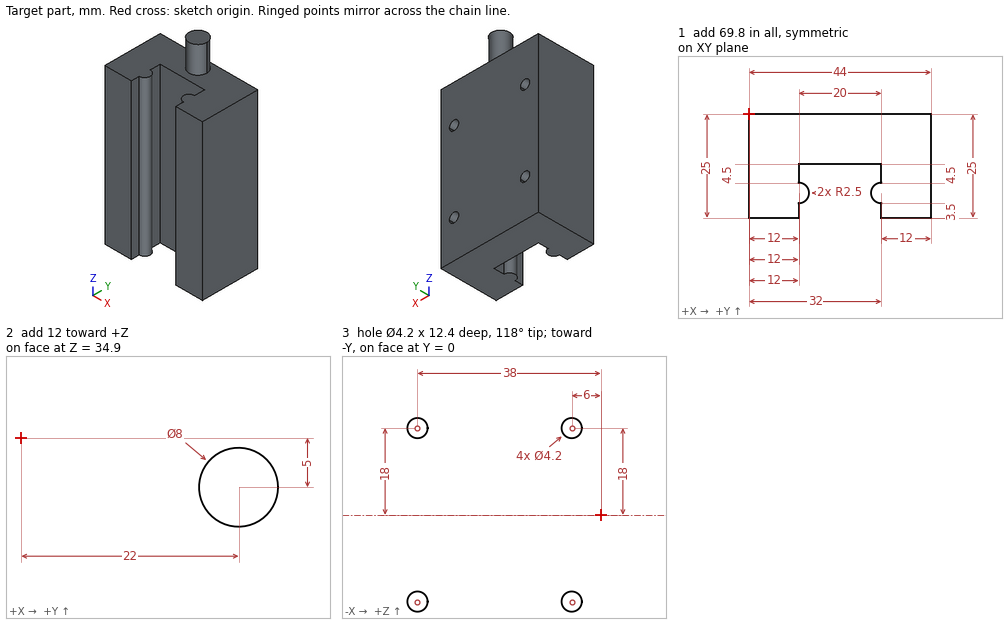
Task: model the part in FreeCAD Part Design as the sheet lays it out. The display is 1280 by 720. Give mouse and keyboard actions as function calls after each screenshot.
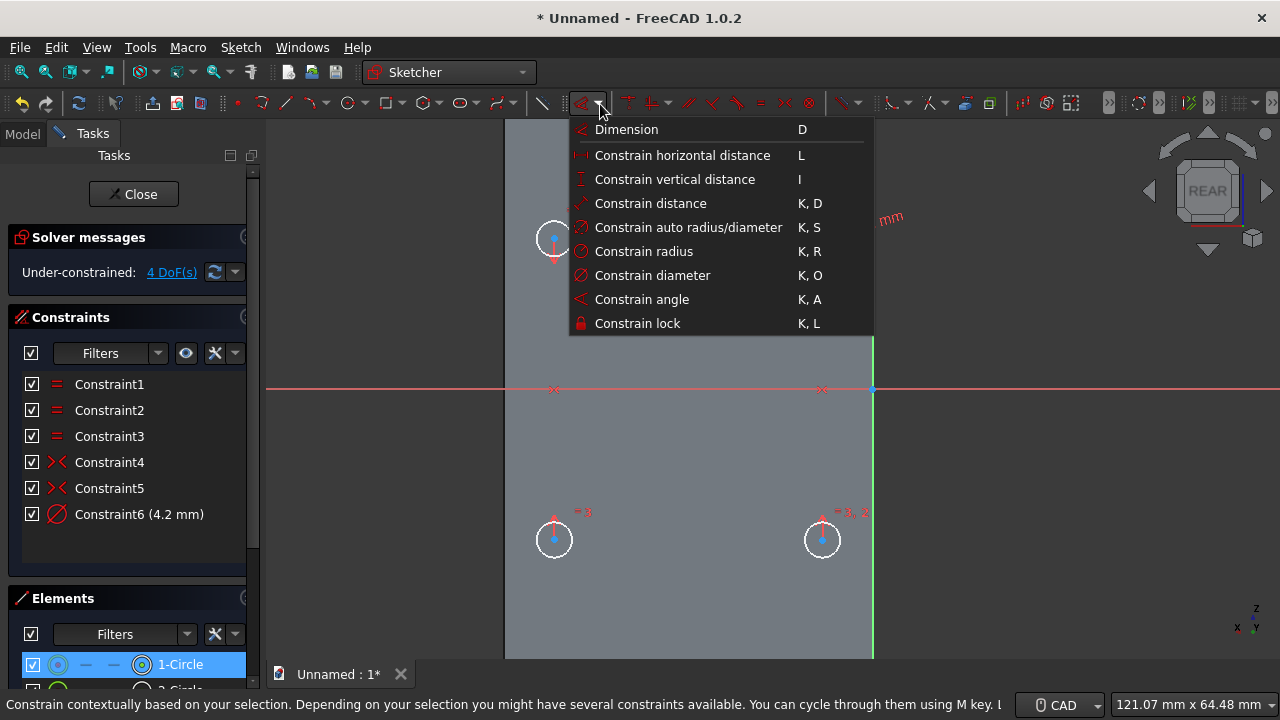
click(722, 155)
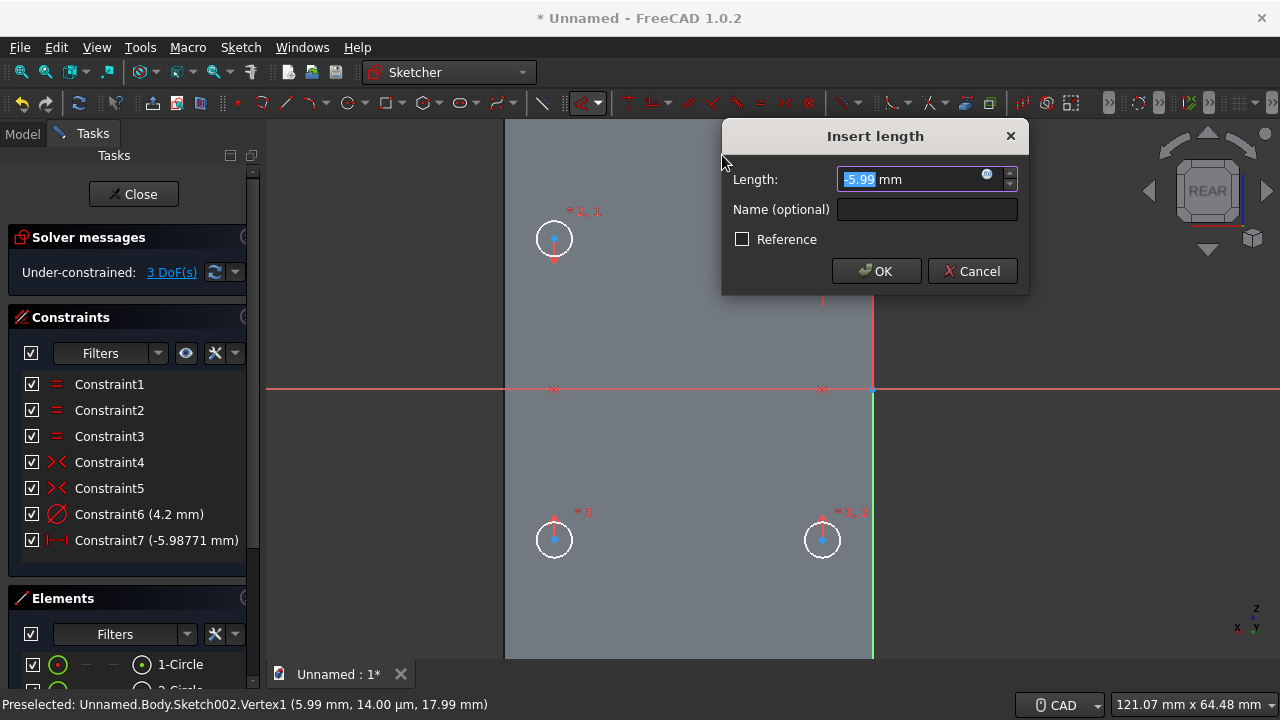
text(-6)
key(Return)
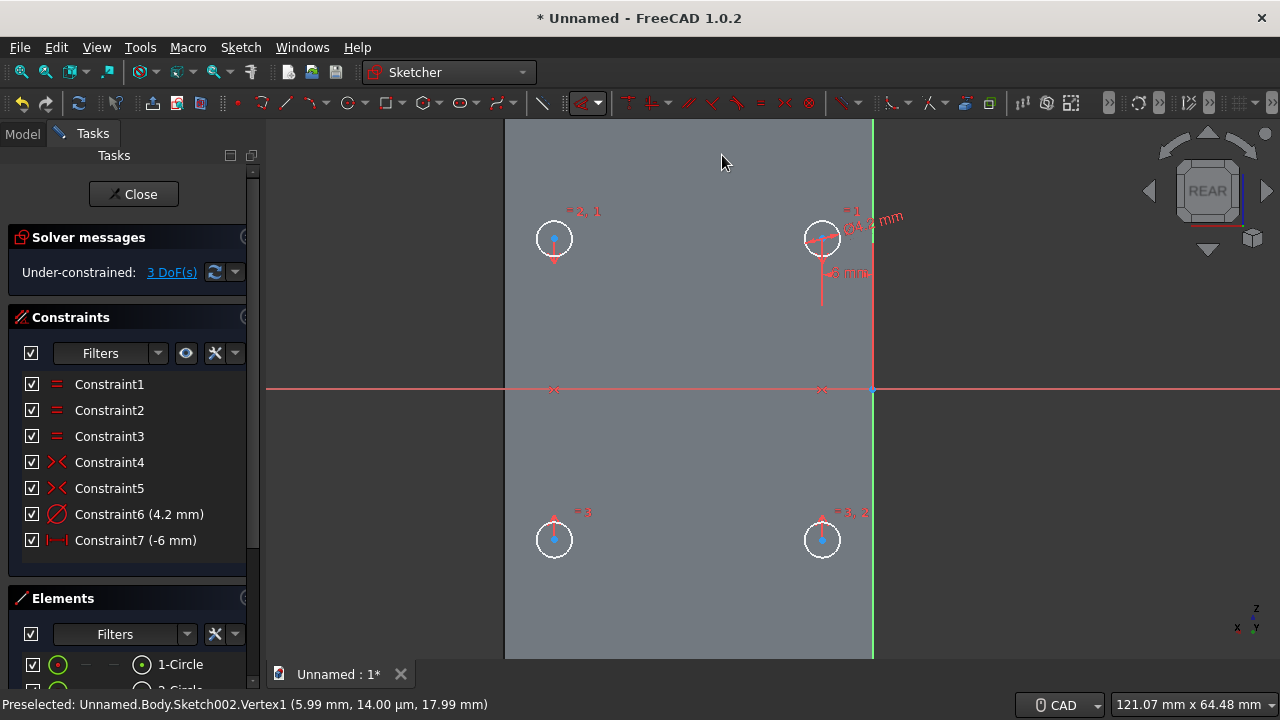
click(822, 239)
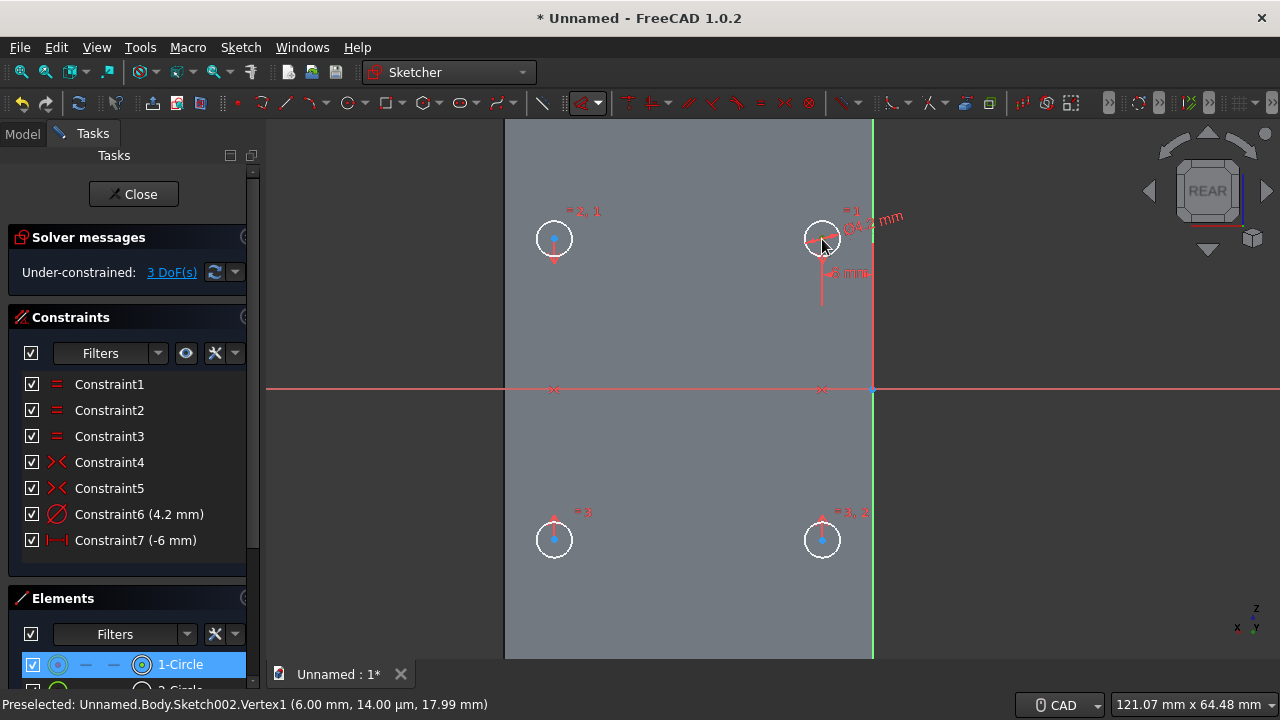
click(600, 104)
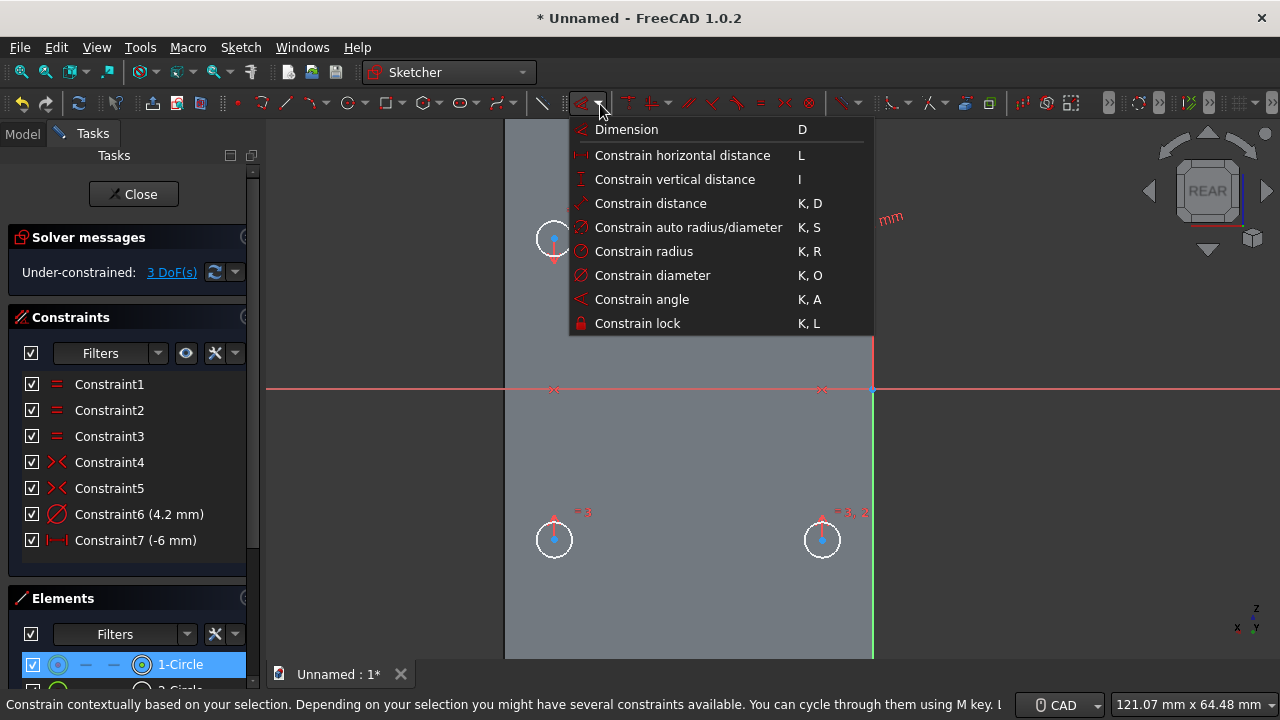
click(722, 179)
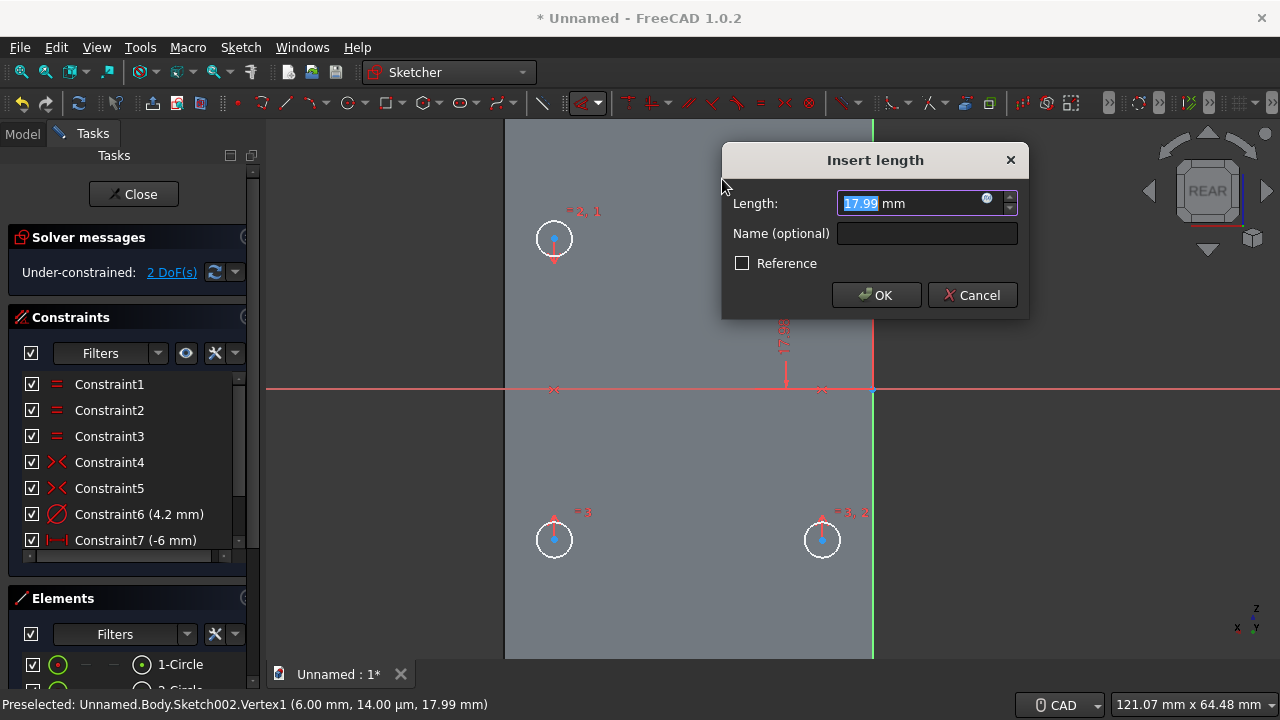
text(18)
key(Return)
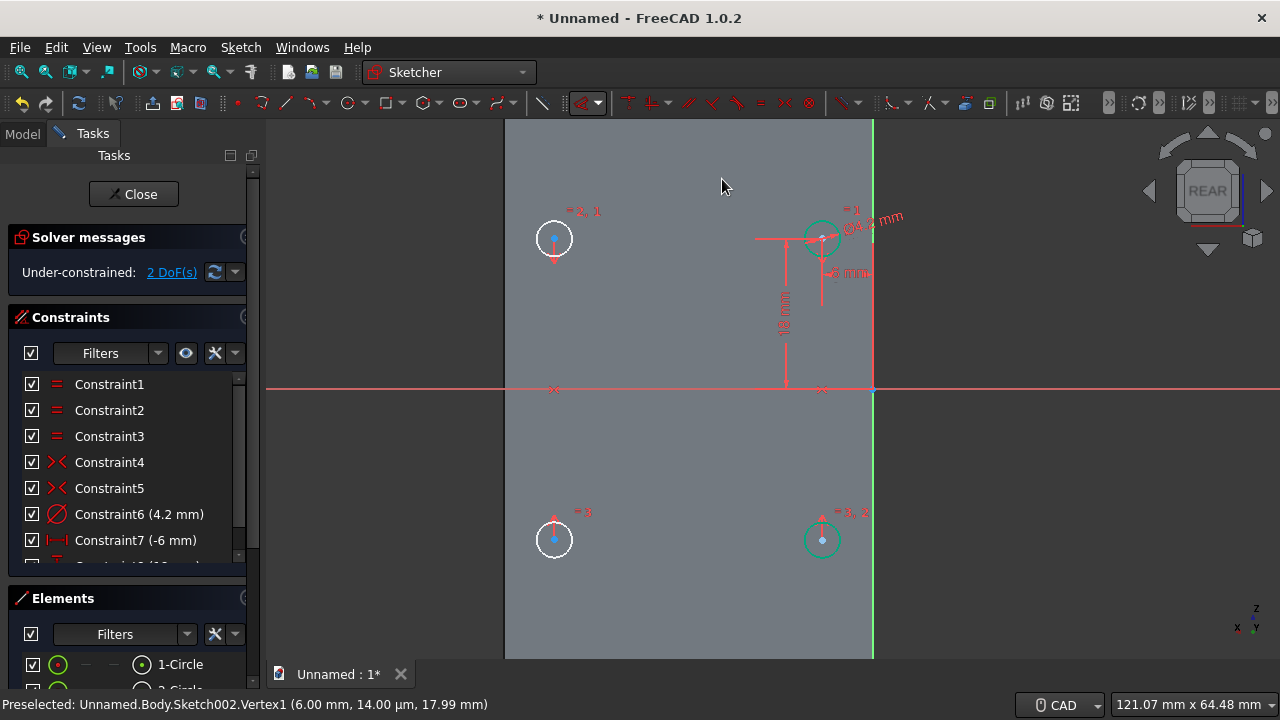
click(554, 239)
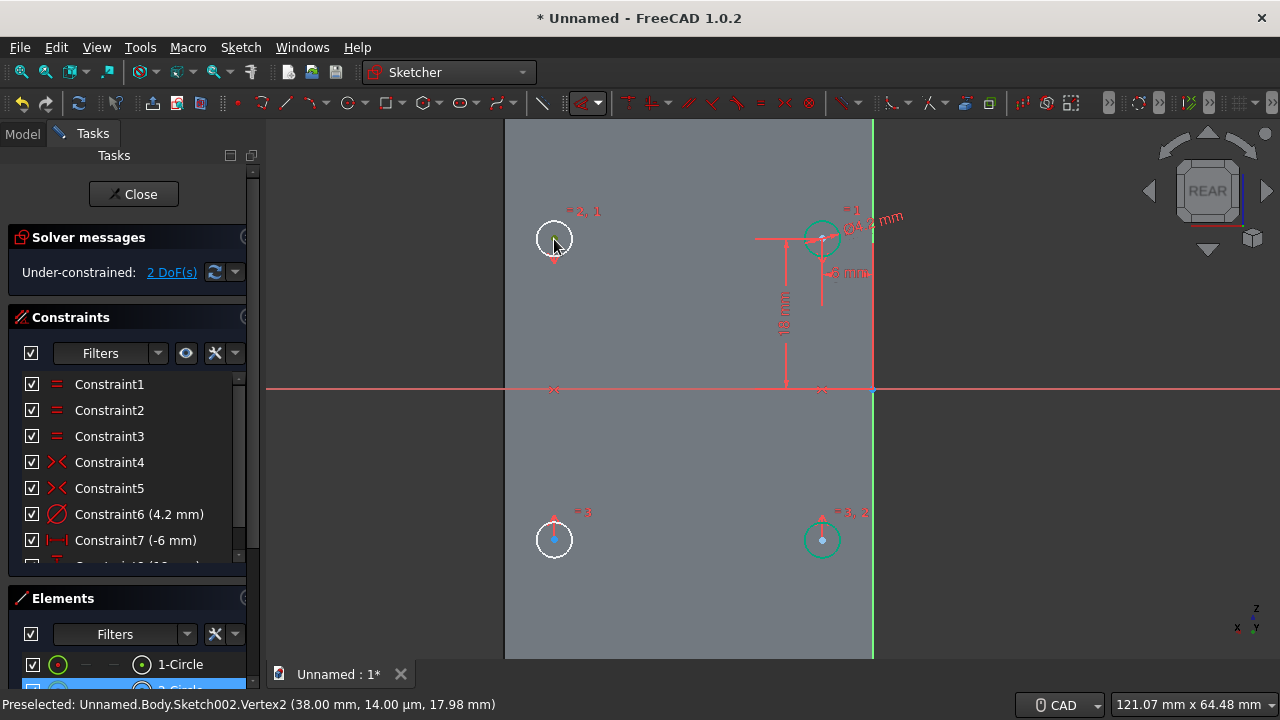
key(l)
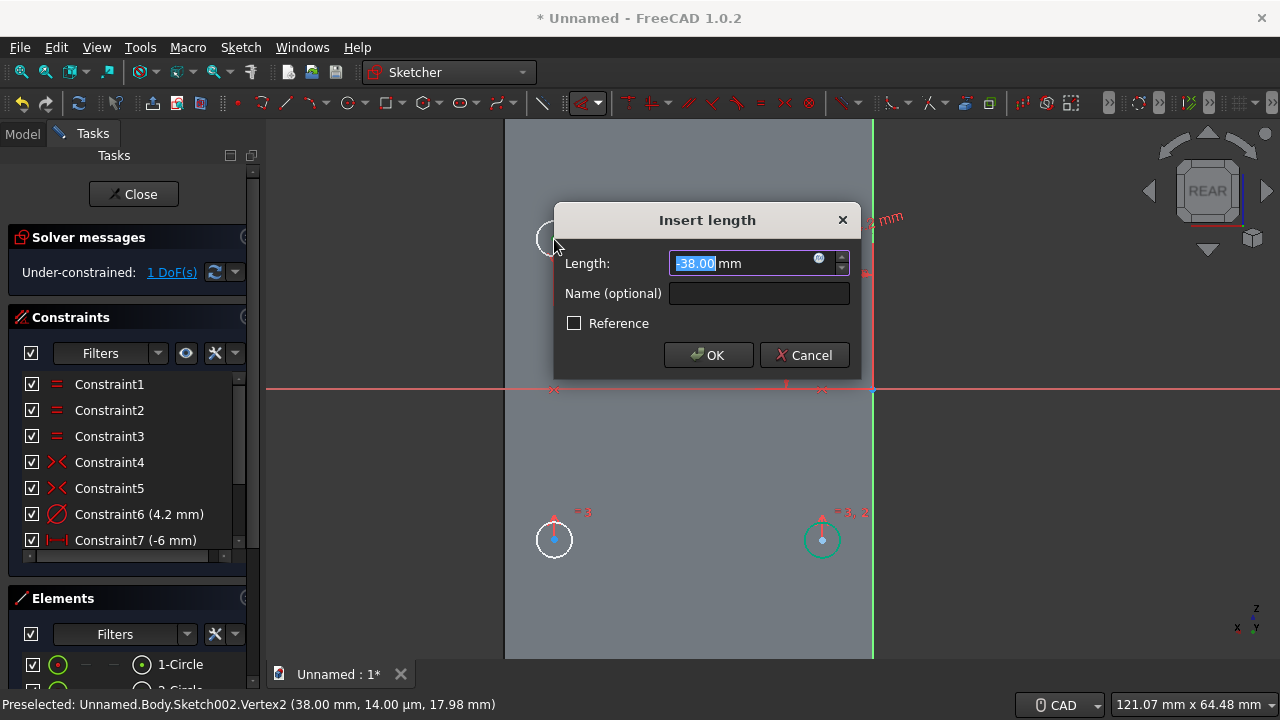
text(-38)
key(Return)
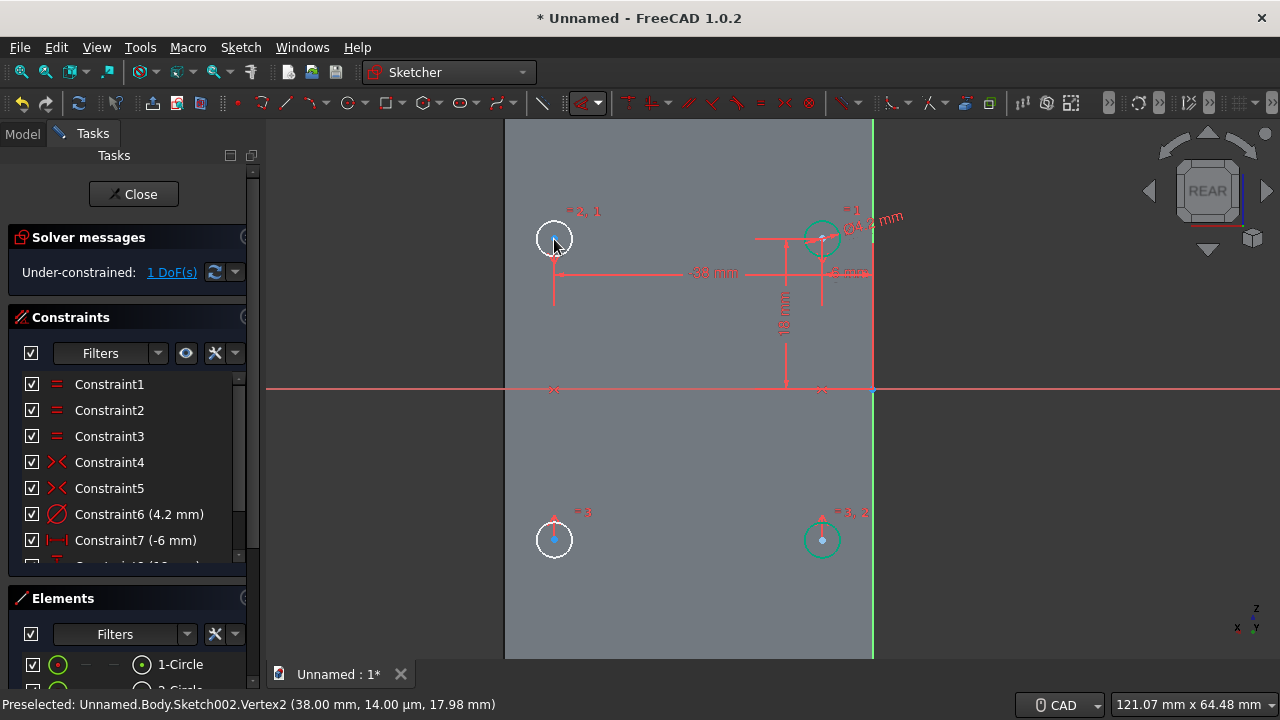
click(554, 239)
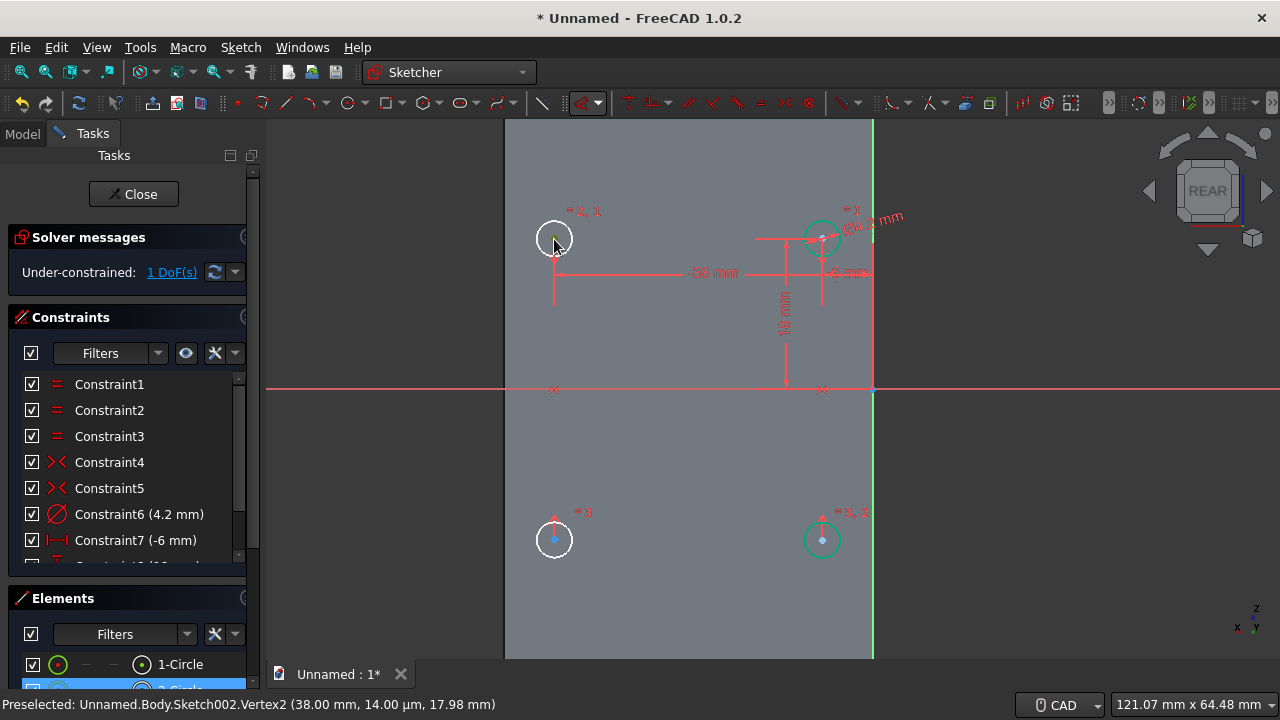
click(600, 104)